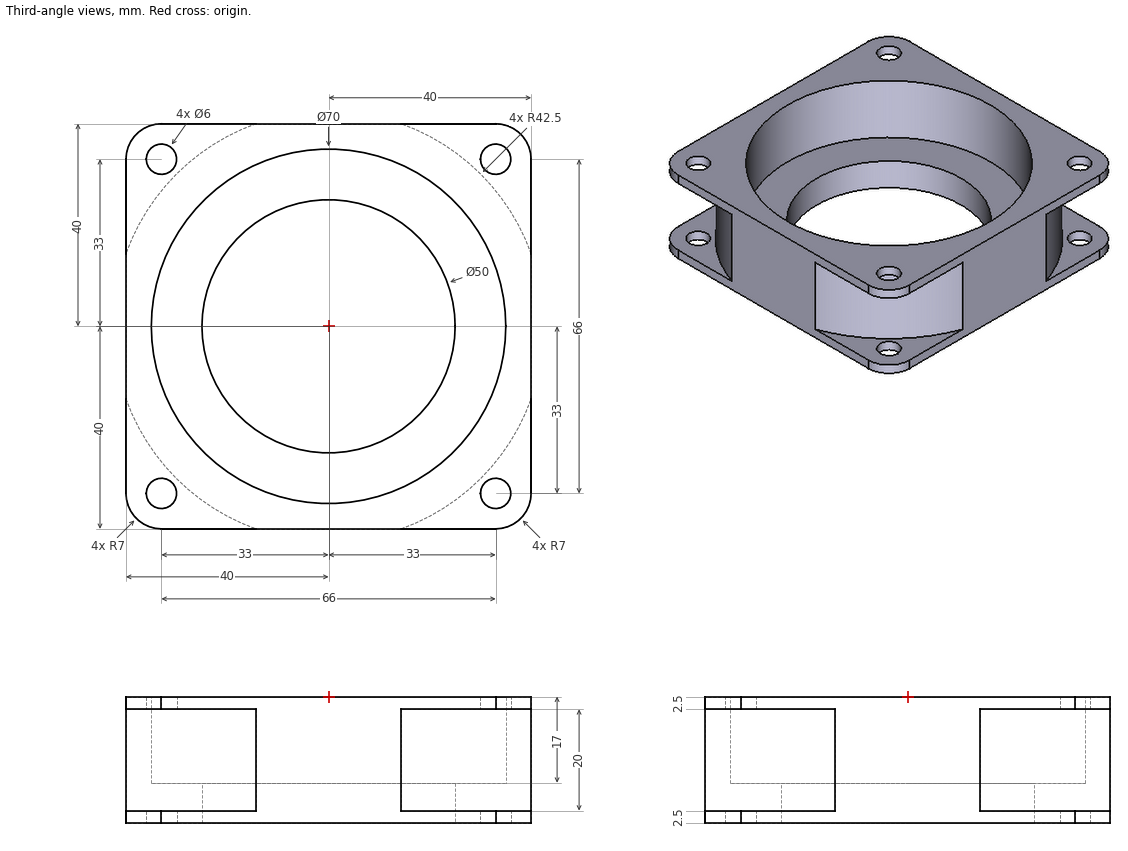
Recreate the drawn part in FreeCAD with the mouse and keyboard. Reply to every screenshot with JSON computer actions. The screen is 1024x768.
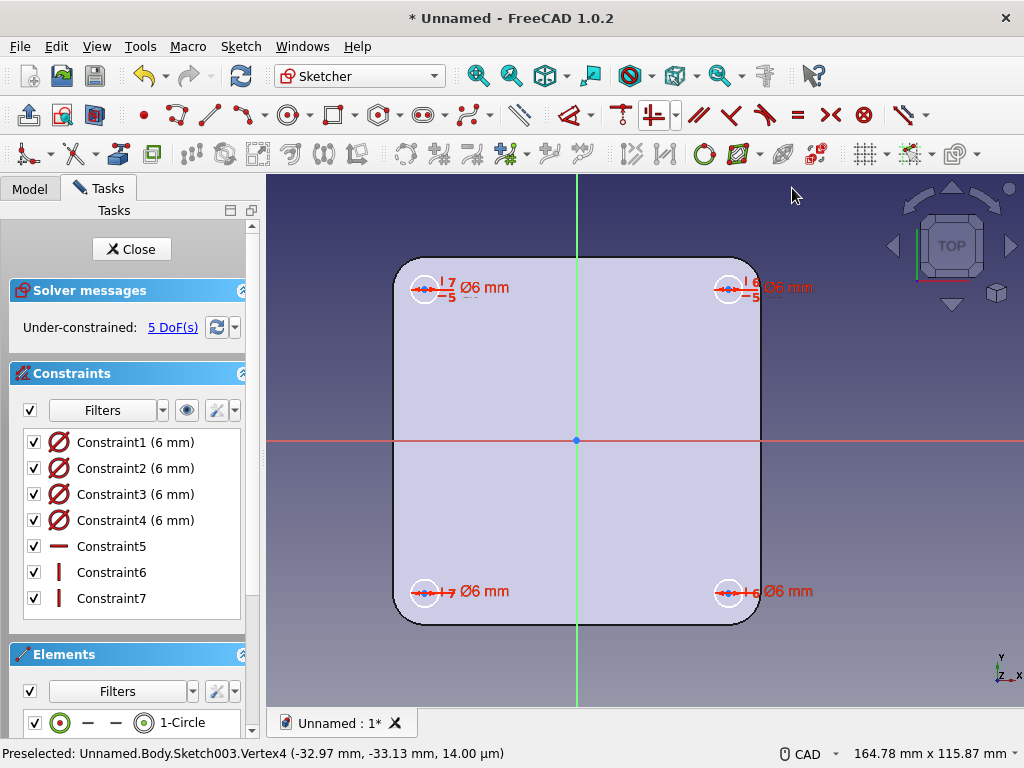
{"action": "left_click", "coordinate": [729, 593]}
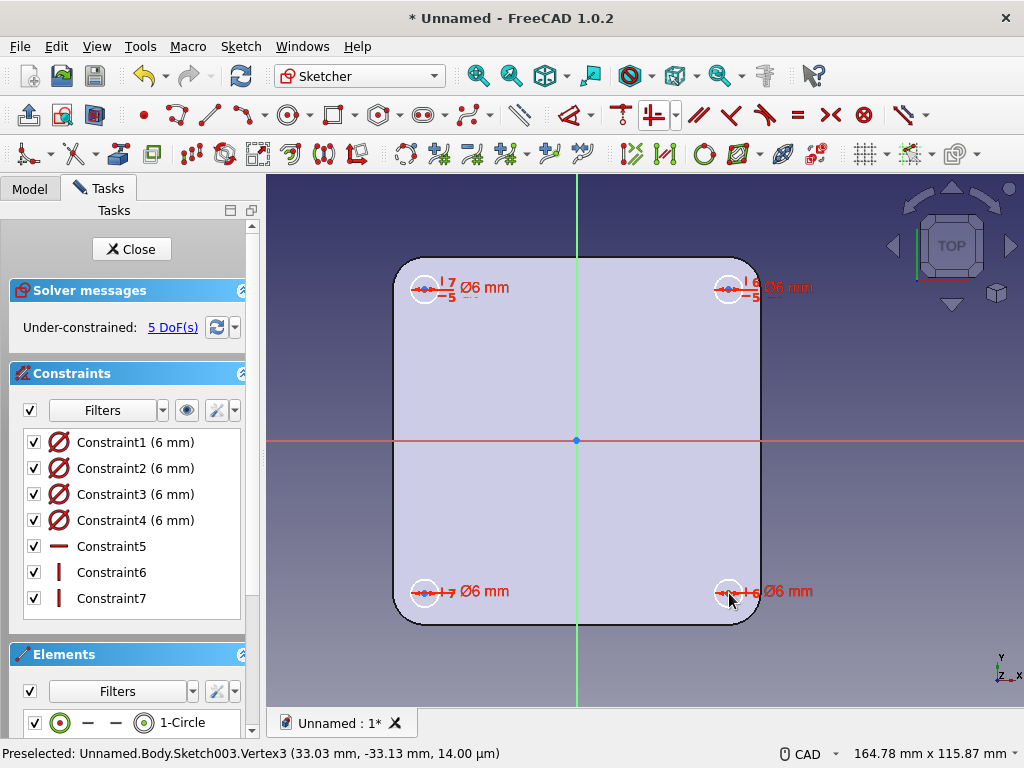
{"action": "left_click", "coordinate": [425, 593]}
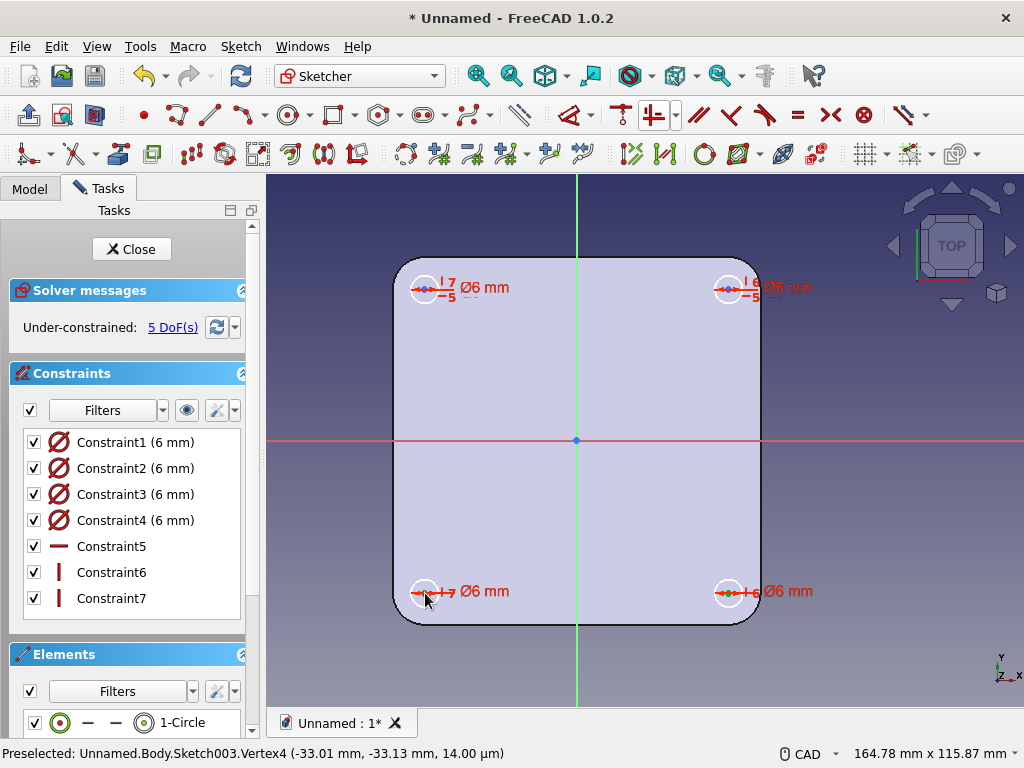
{"action": "left_click", "coordinate": [676, 116]}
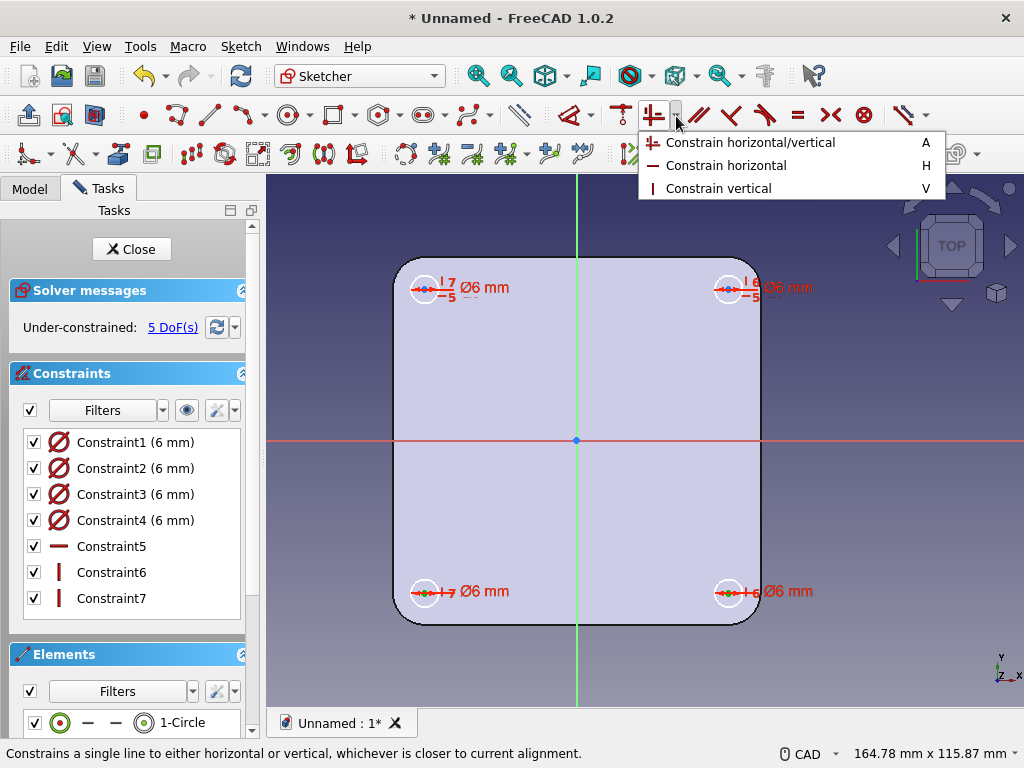
{"action": "left_click", "coordinate": [792, 166]}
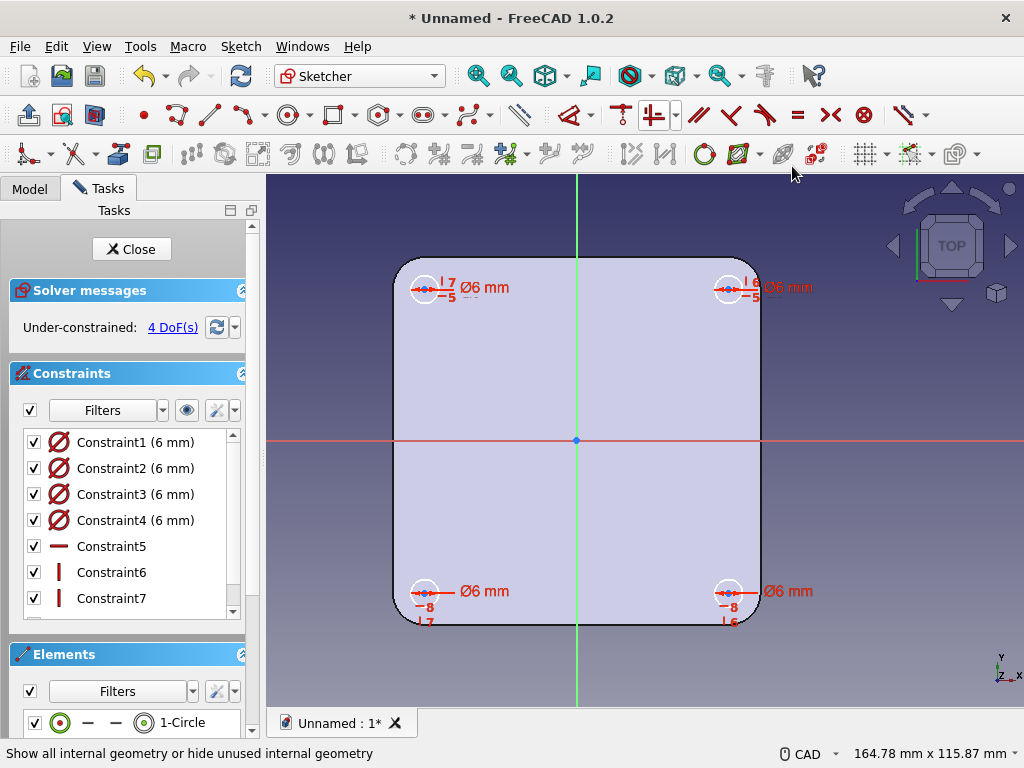
{"action": "left_click", "coordinate": [568, 116]}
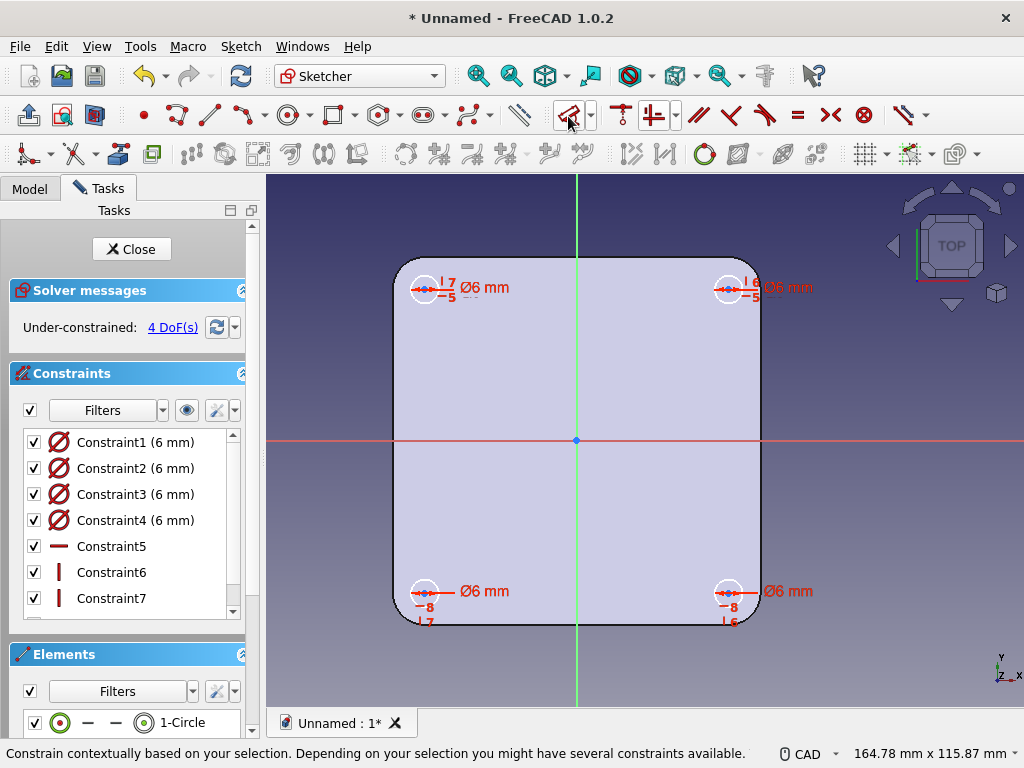
{"action": "left_click", "coordinate": [425, 290]}
{"action": "left_click", "coordinate": [501, 256]}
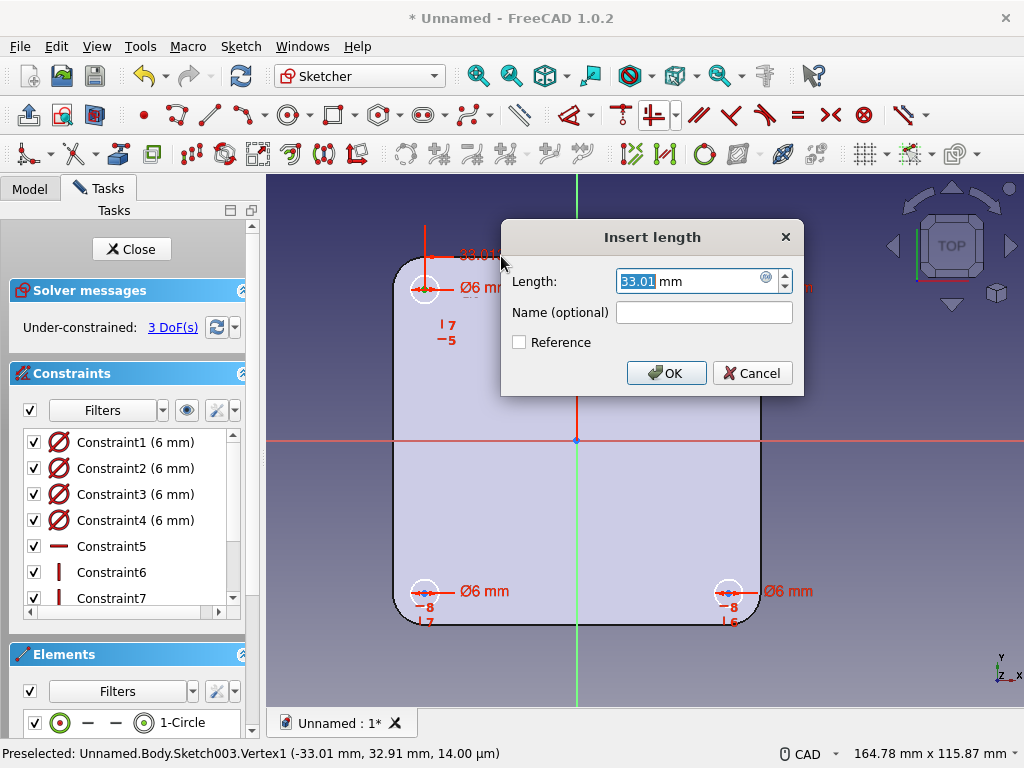
{"action": "type", "text": "33"}
{"action": "key", "text": "Return"}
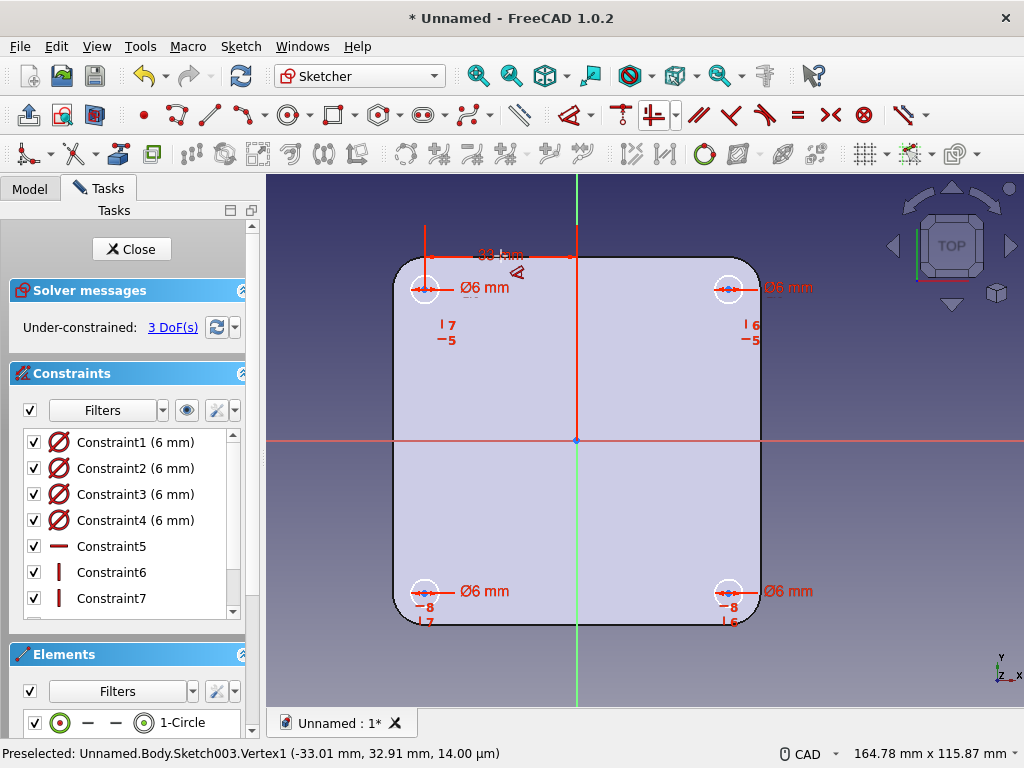
{"action": "left_click", "coordinate": [425, 290]}
{"action": "left_click", "coordinate": [391, 365]}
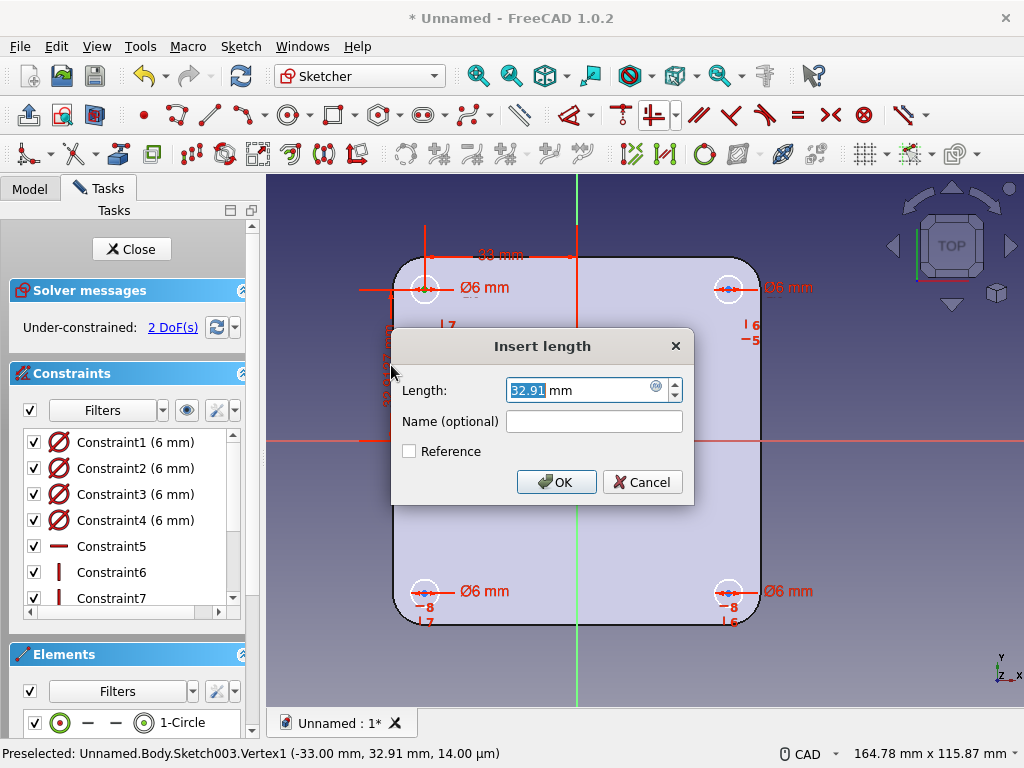
{"action": "type", "text": "33"}
{"action": "key", "text": "Return"}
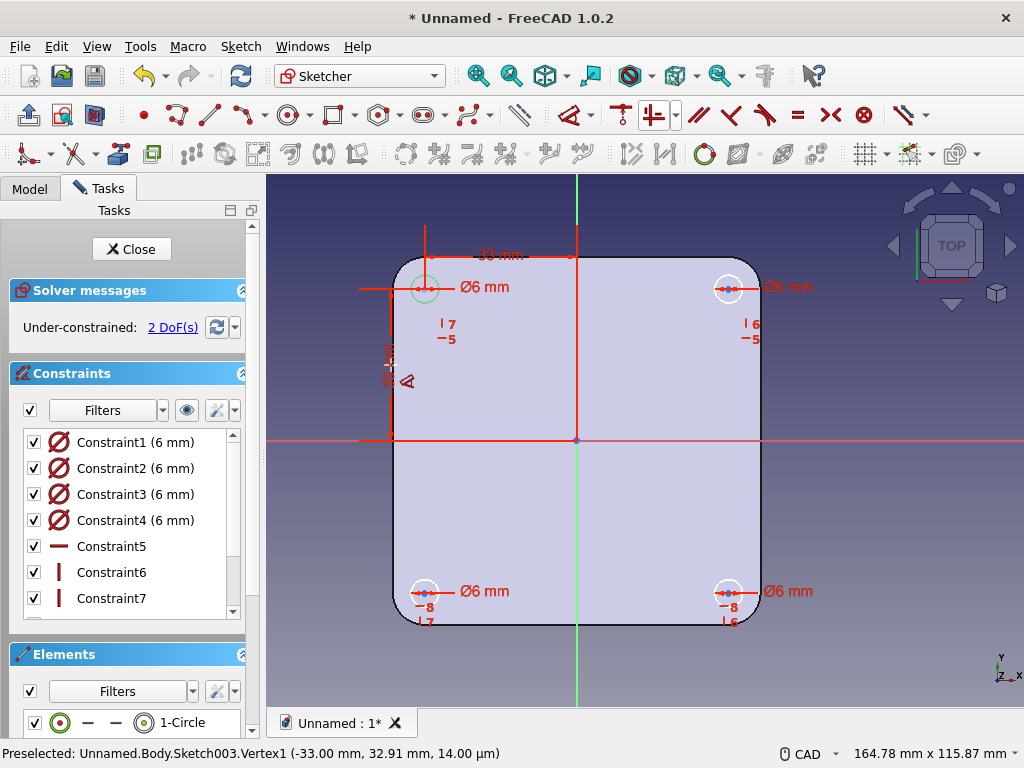
{"action": "left_click", "coordinate": [729, 289]}
{"action": "left_click", "coordinate": [653, 255]}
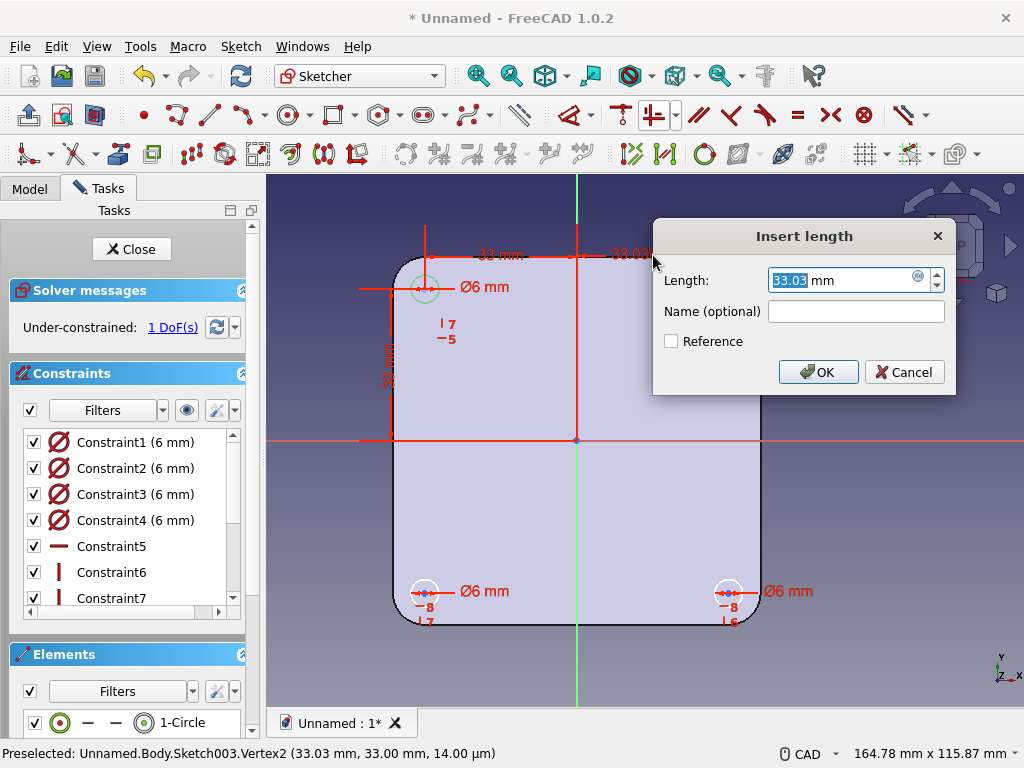
{"action": "type", "text": "33"}
{"action": "key", "text": "Return"}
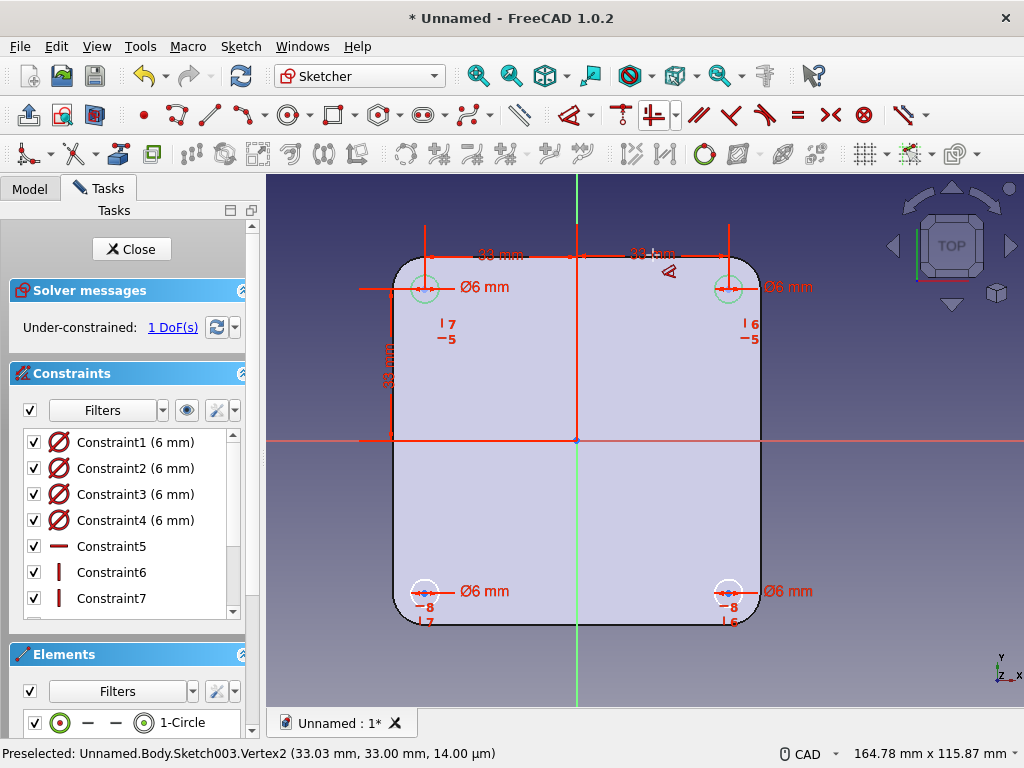
{"action": "left_click", "coordinate": [729, 593]}
{"action": "left_click", "coordinate": [763, 517]}